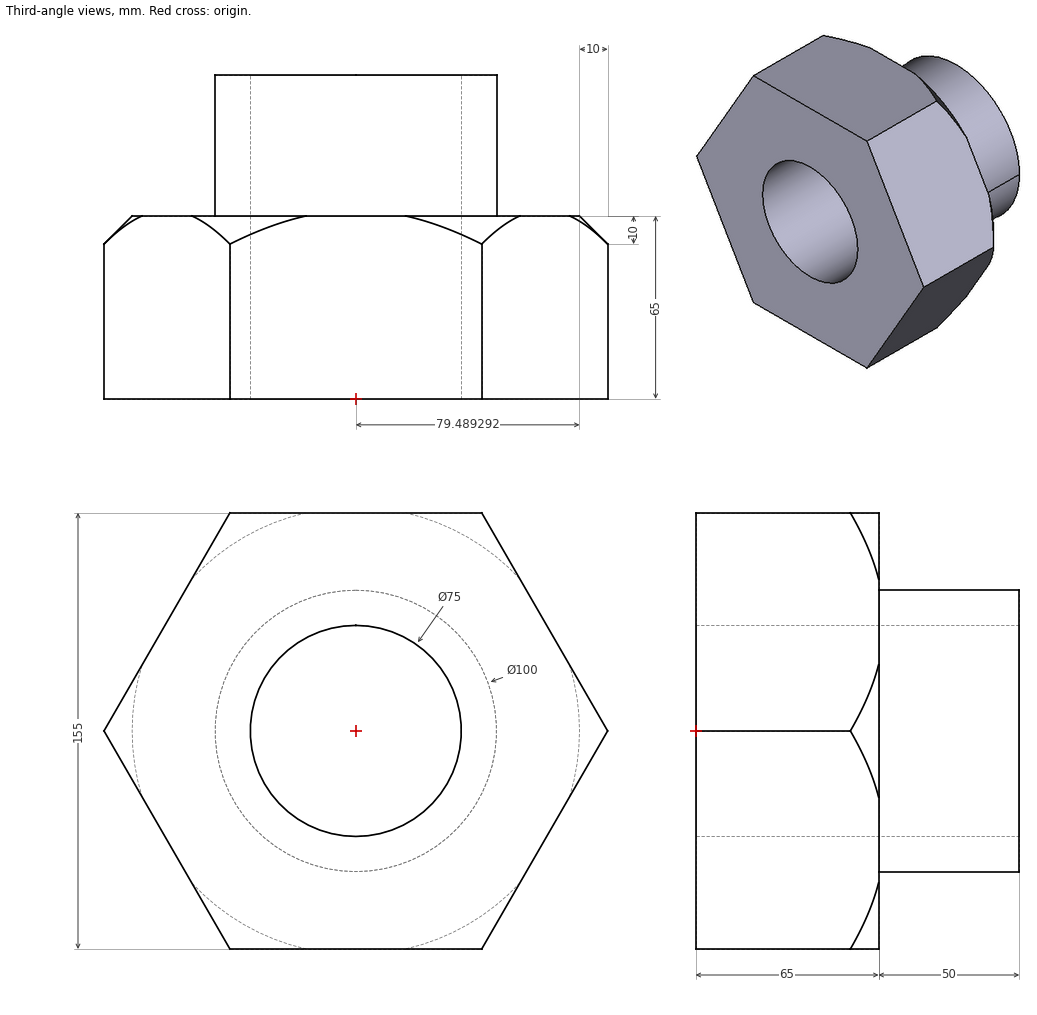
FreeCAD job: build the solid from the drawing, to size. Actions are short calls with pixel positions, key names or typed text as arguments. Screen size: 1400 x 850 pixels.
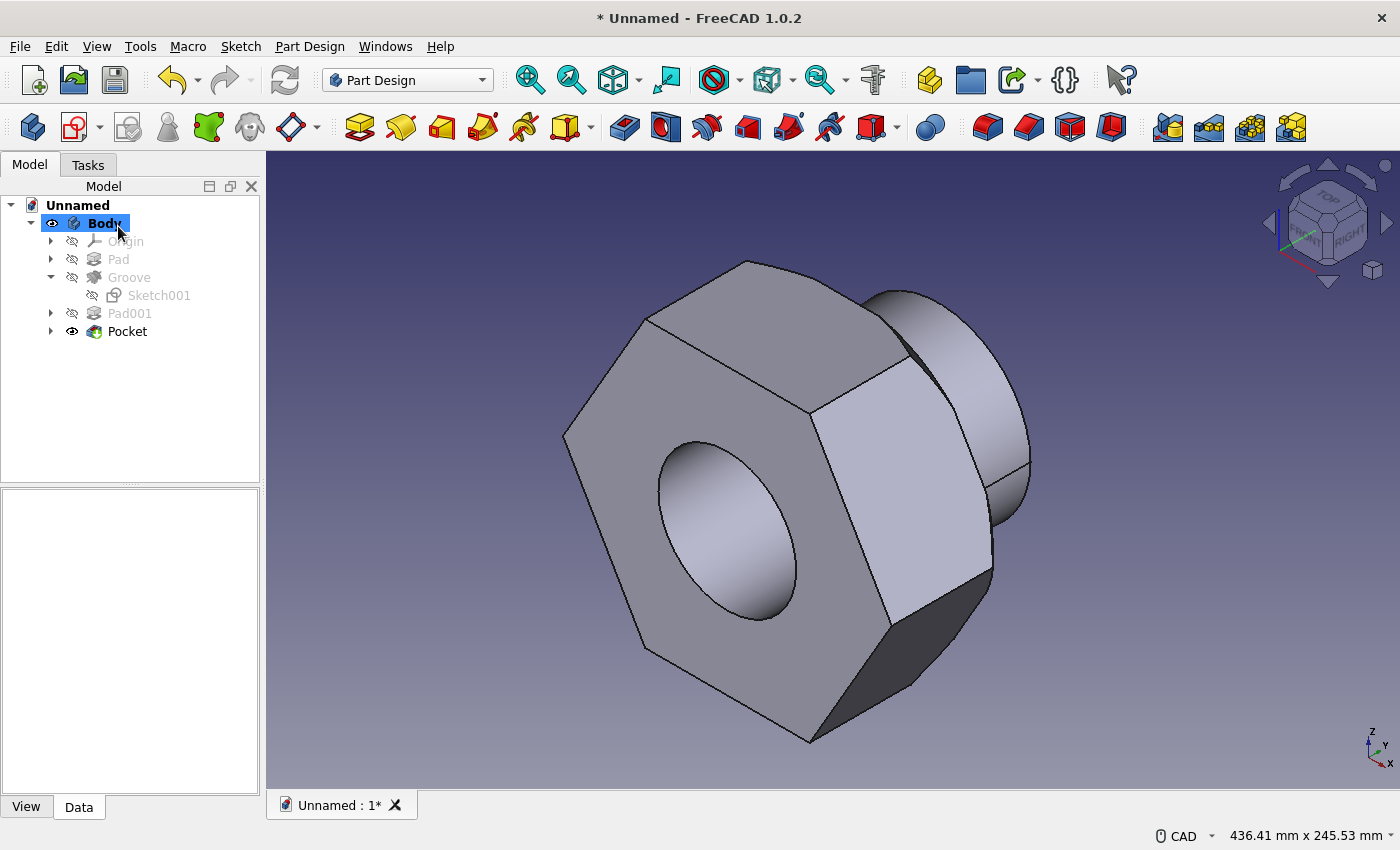
click(531, 80)